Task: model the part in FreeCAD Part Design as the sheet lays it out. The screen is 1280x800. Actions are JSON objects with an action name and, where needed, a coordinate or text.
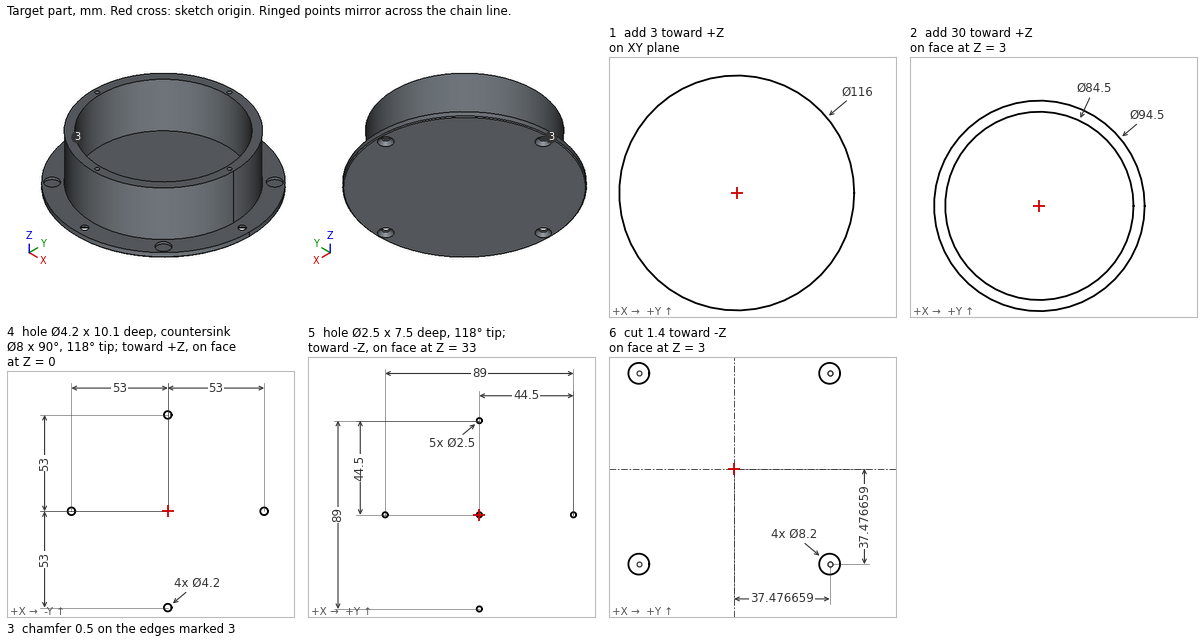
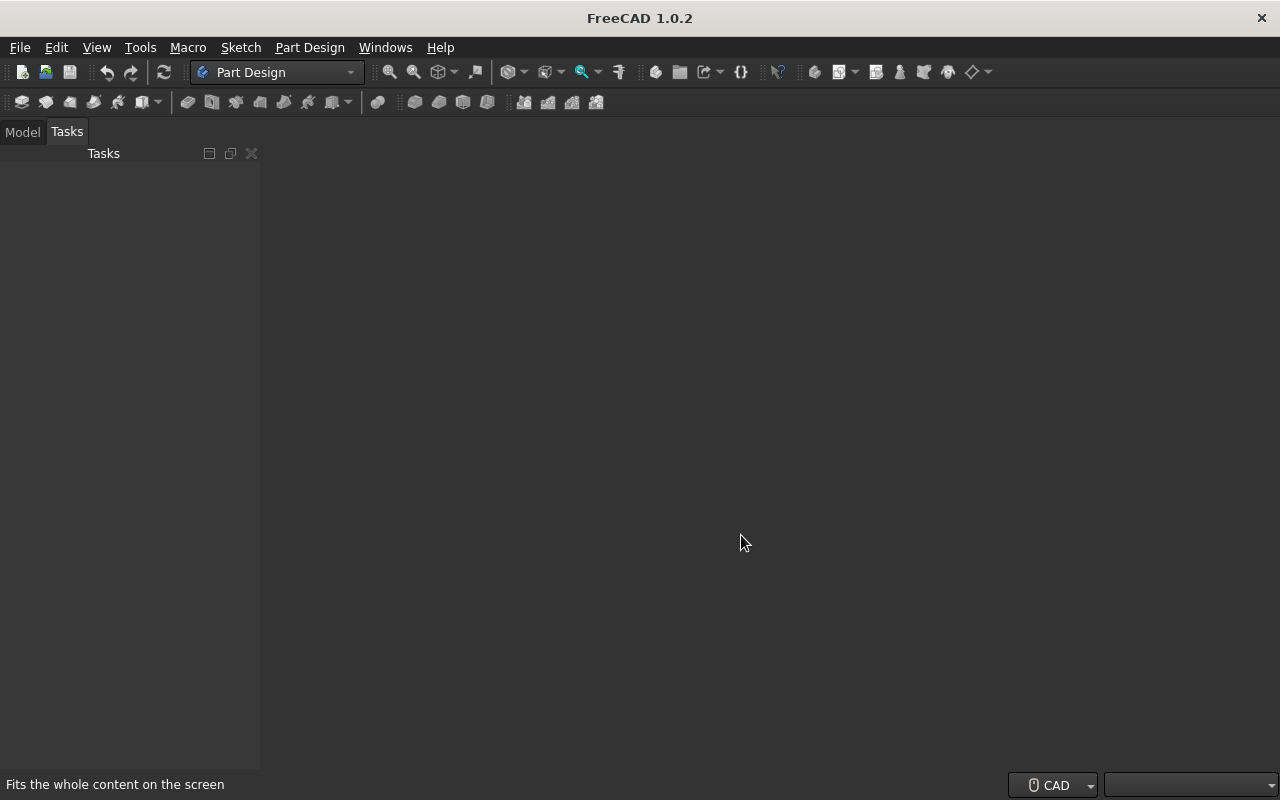
{"action": "left_click", "coordinate": [22, 72]}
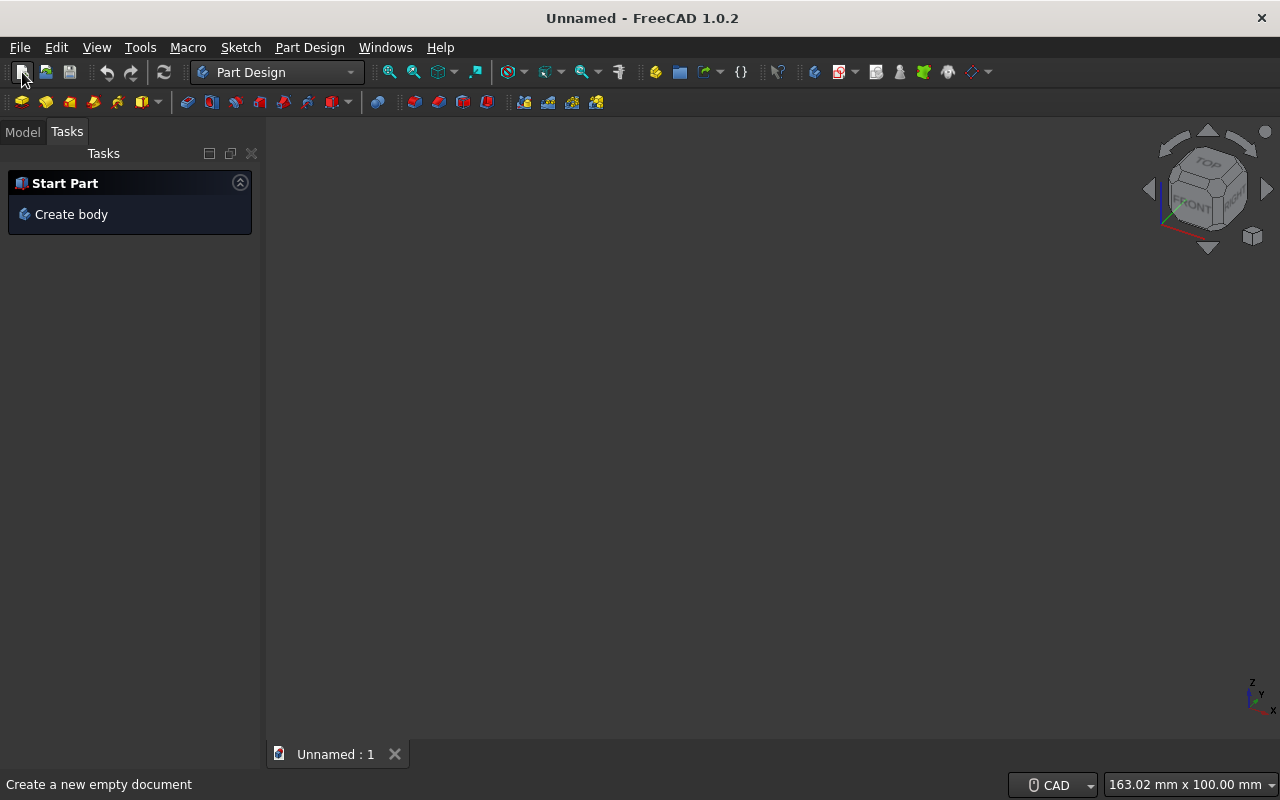
{"action": "left_click", "coordinate": [840, 72]}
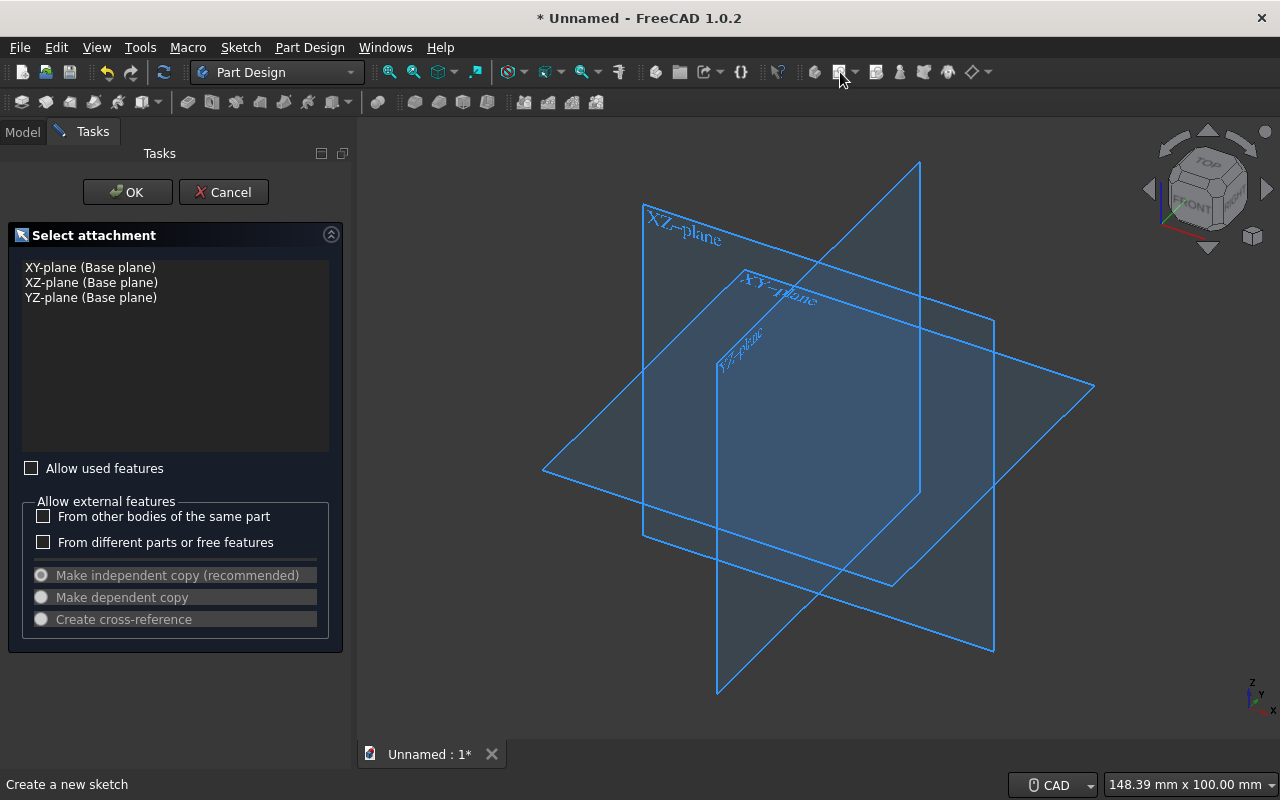
{"action": "left_click", "coordinate": [82, 268]}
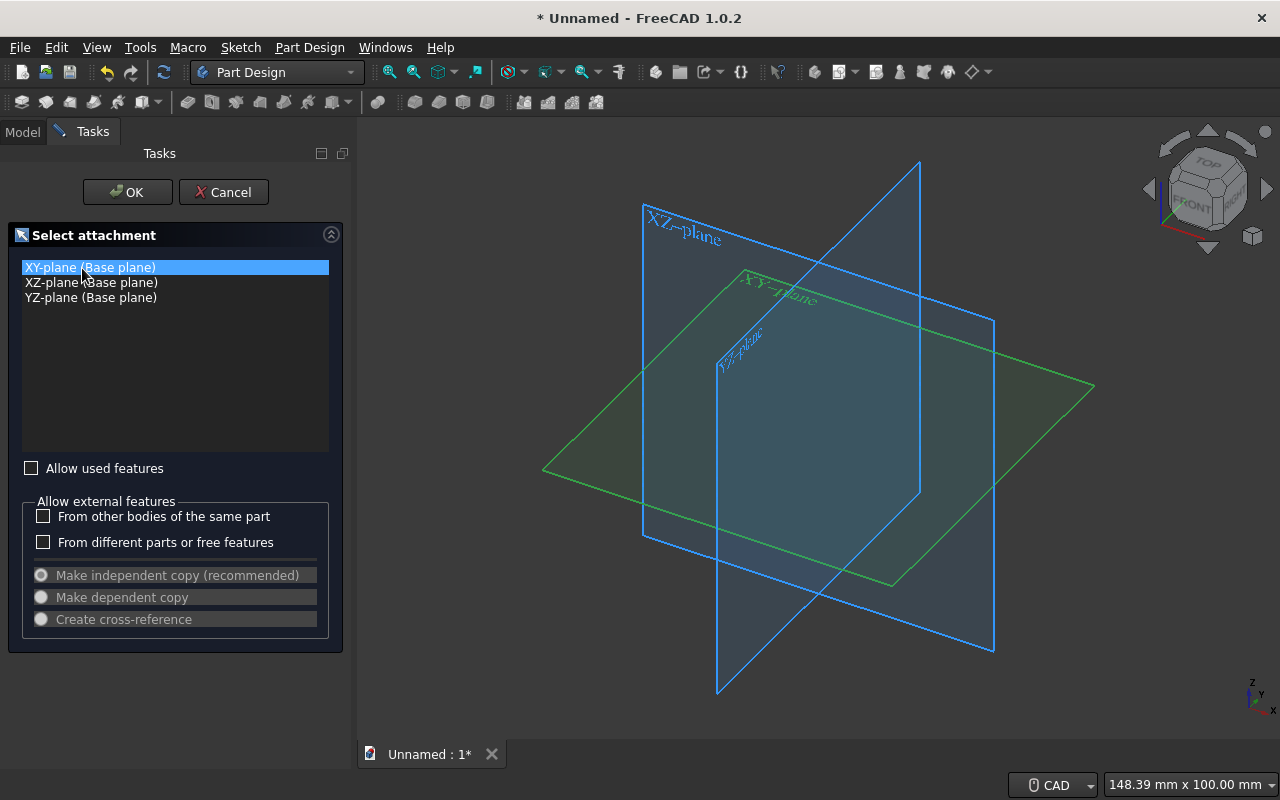
{"action": "left_click", "coordinate": [128, 192]}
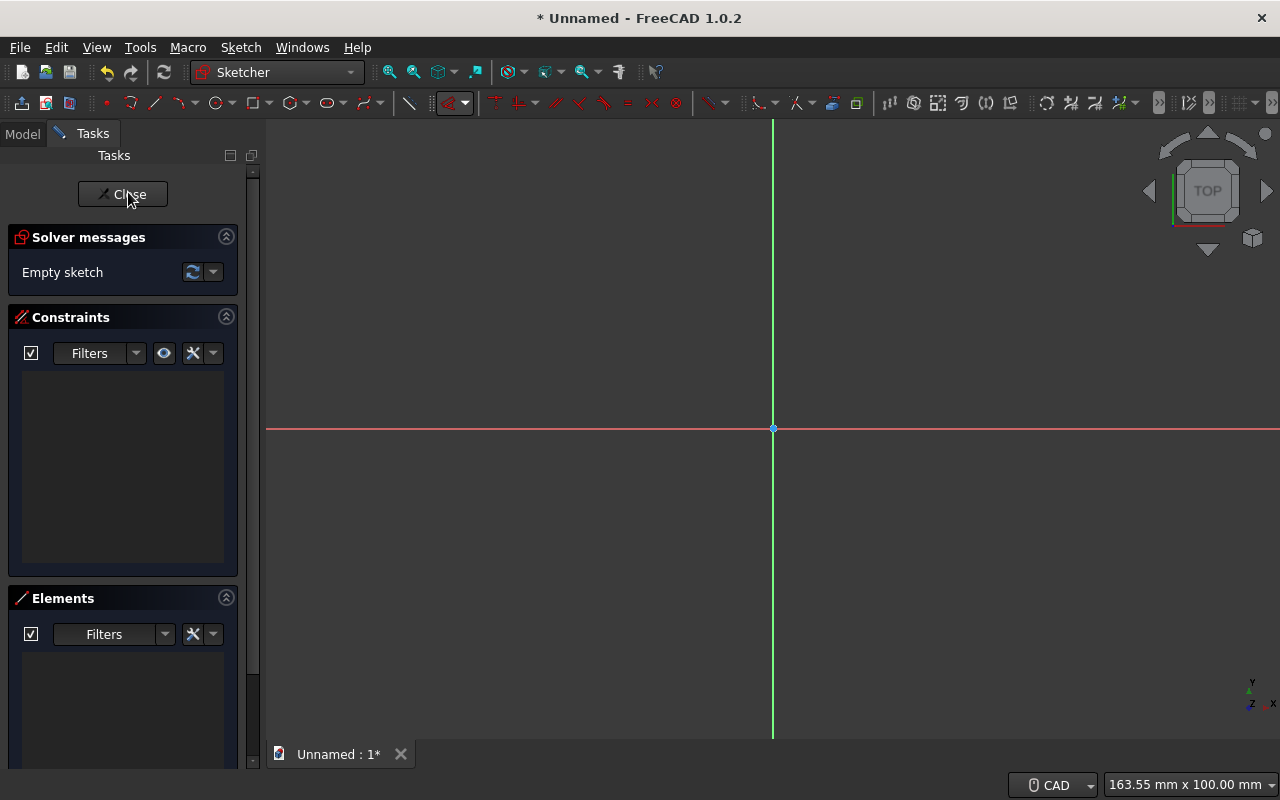
{"action": "scroll", "coordinate": [621, 429], "scroll_direction": "down", "scroll_amount": 3}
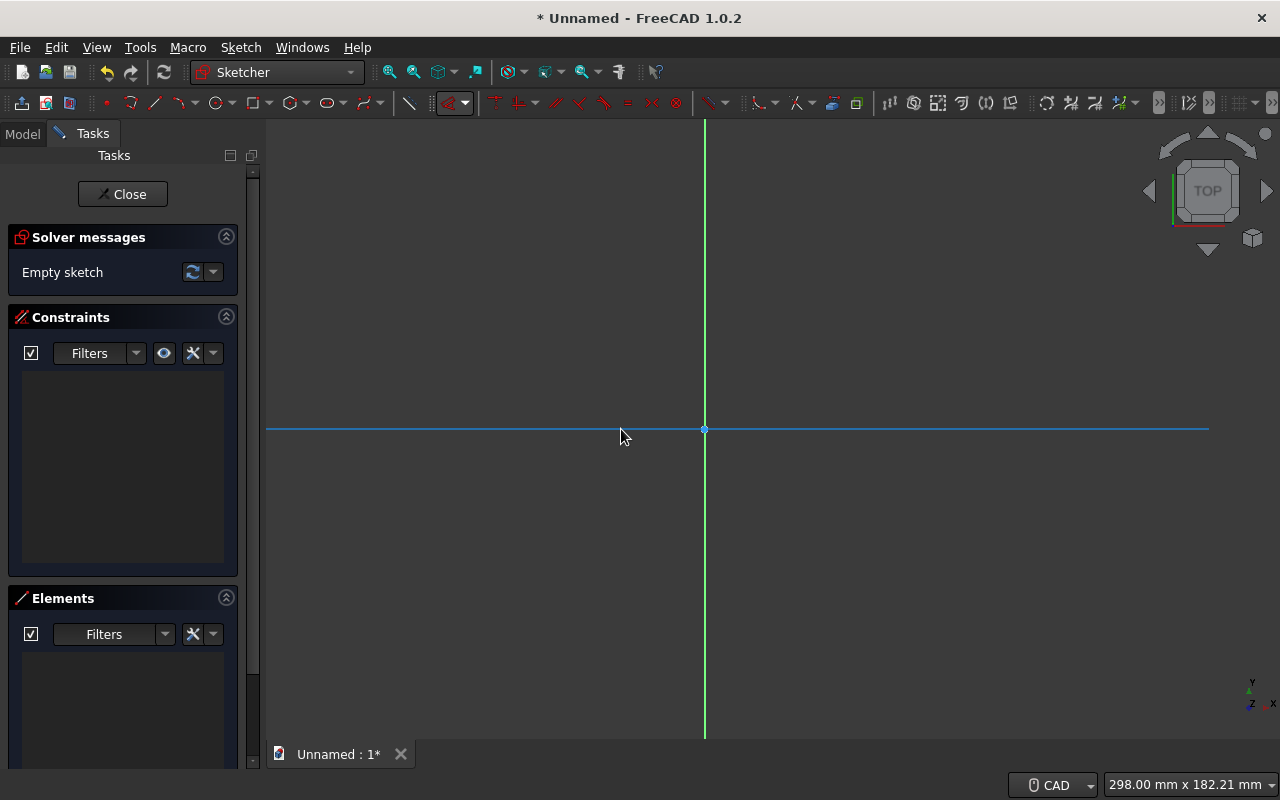
{"action": "left_click", "coordinate": [216, 104]}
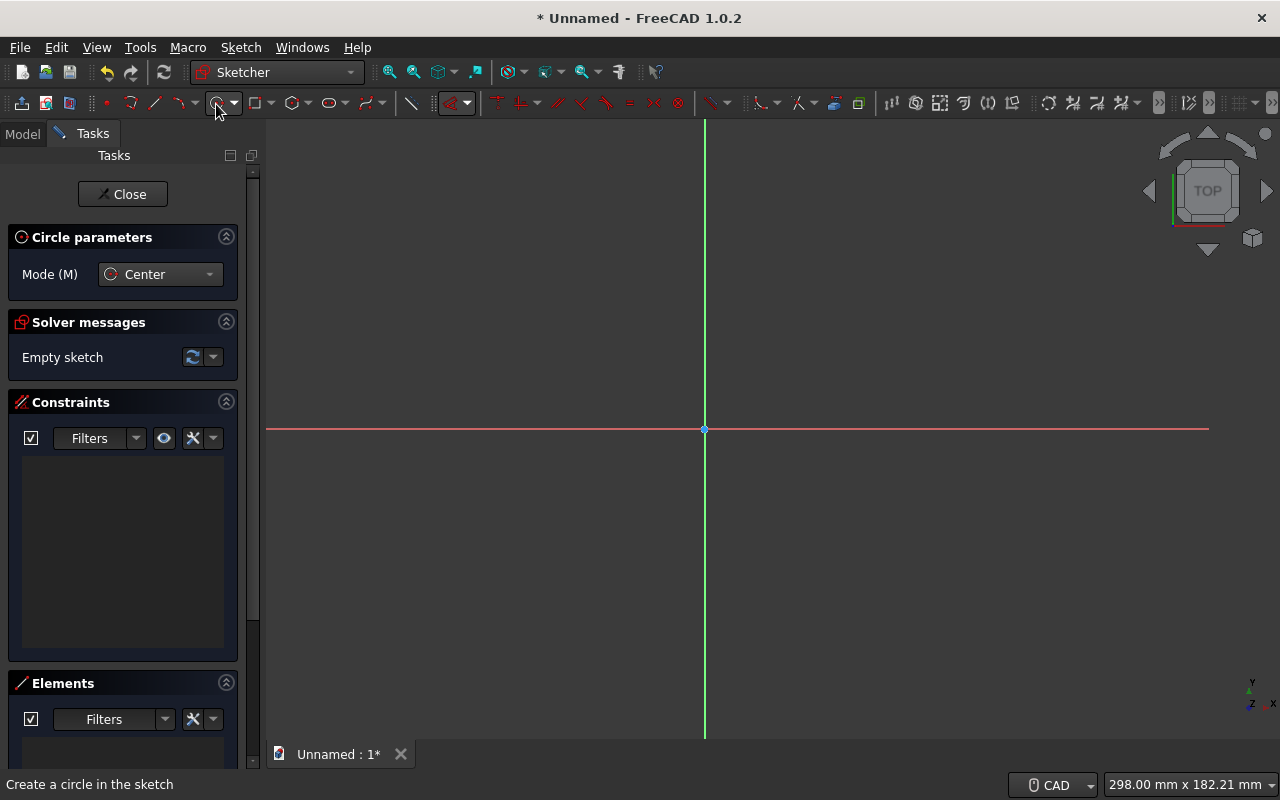
{"action": "left_click", "coordinate": [705, 429]}
{"action": "mouse_move", "coordinate": [844, 290]}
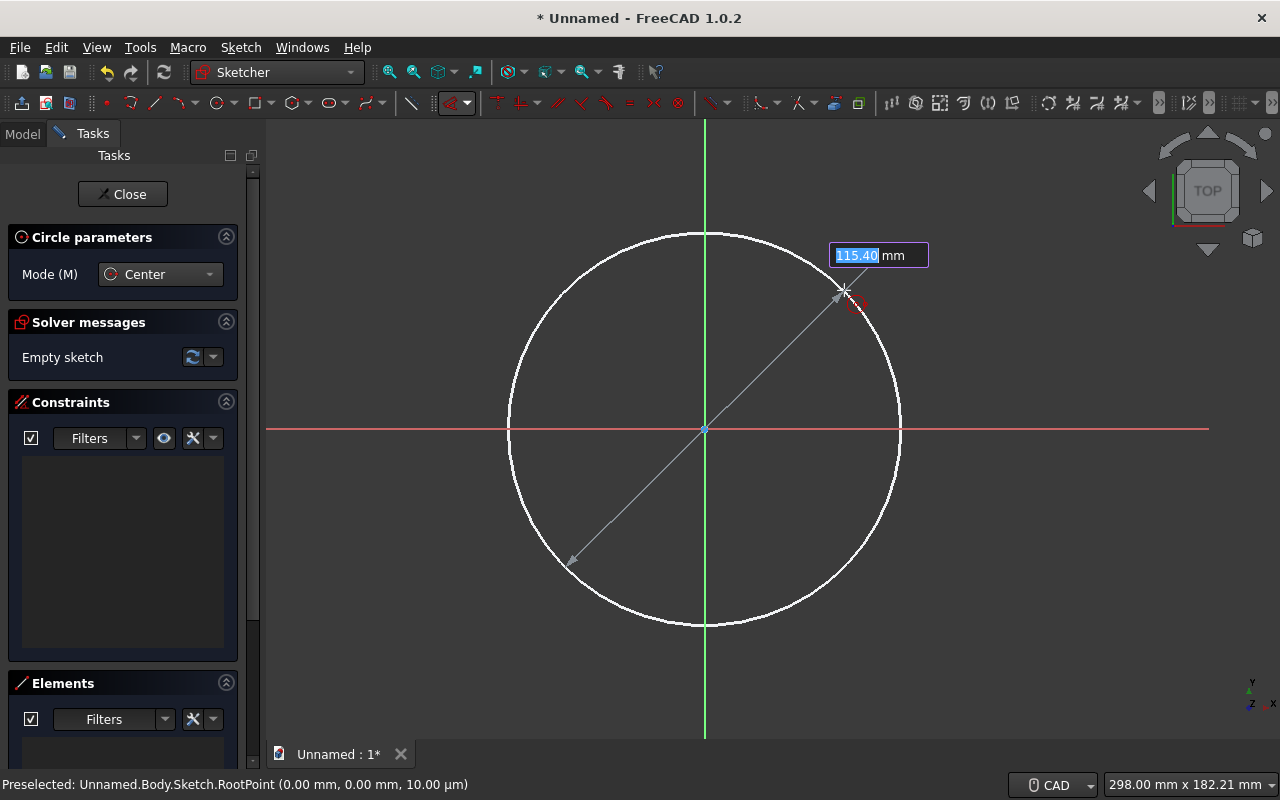
{"action": "type", "text": "116"}
{"action": "key", "text": "Return"}
{"action": "key", "text": "Escape"}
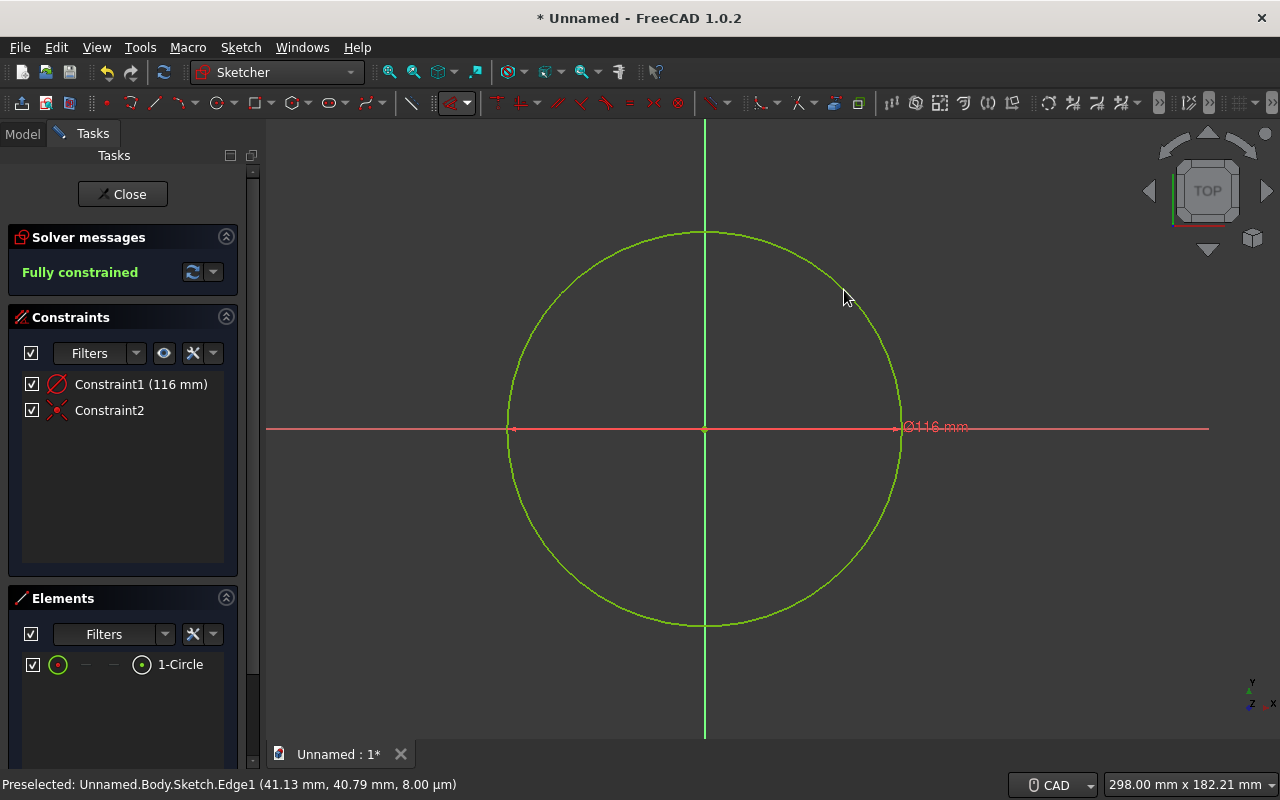
{"action": "left_click", "coordinate": [123, 194]}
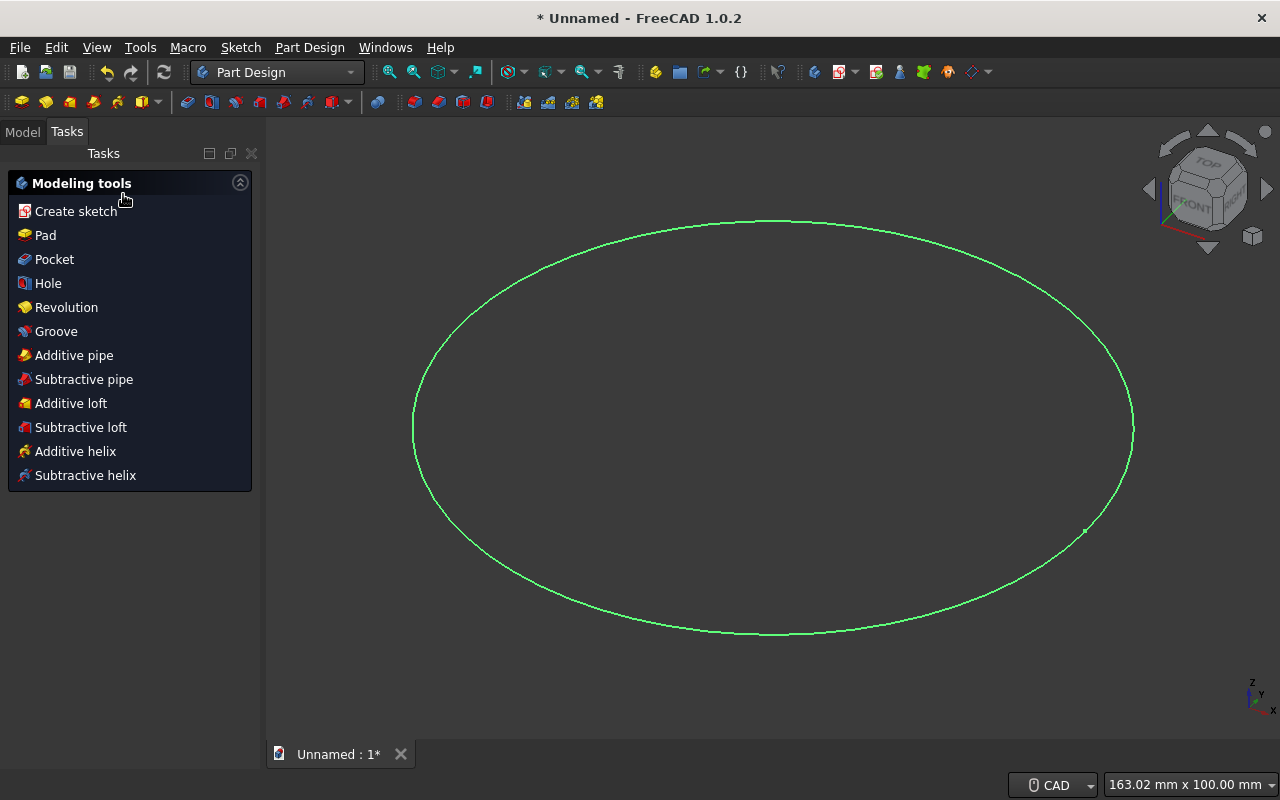
{"action": "left_click", "coordinate": [22, 102]}